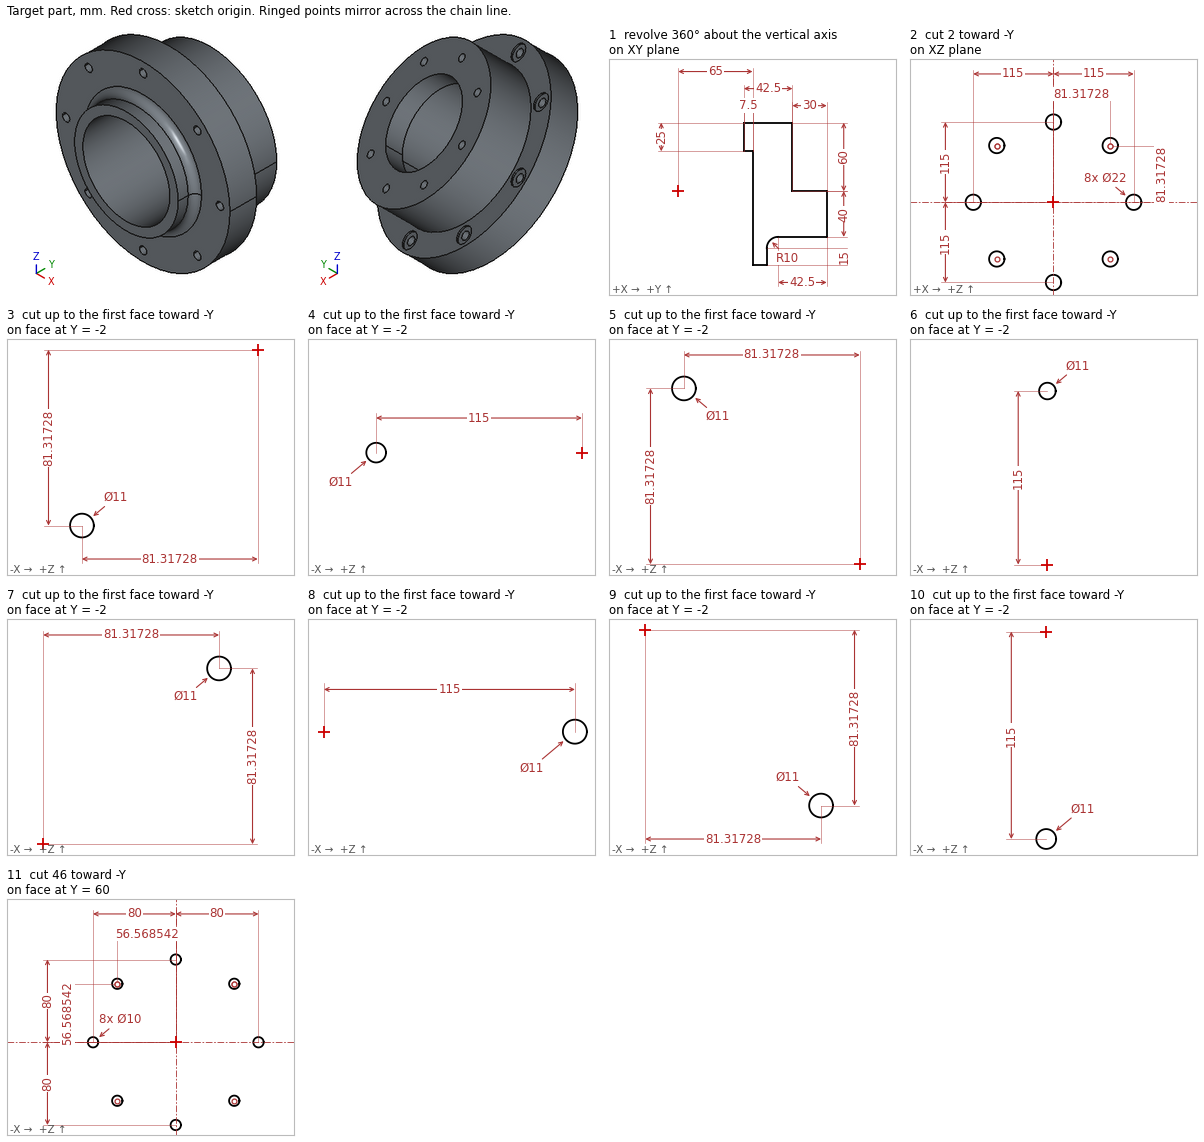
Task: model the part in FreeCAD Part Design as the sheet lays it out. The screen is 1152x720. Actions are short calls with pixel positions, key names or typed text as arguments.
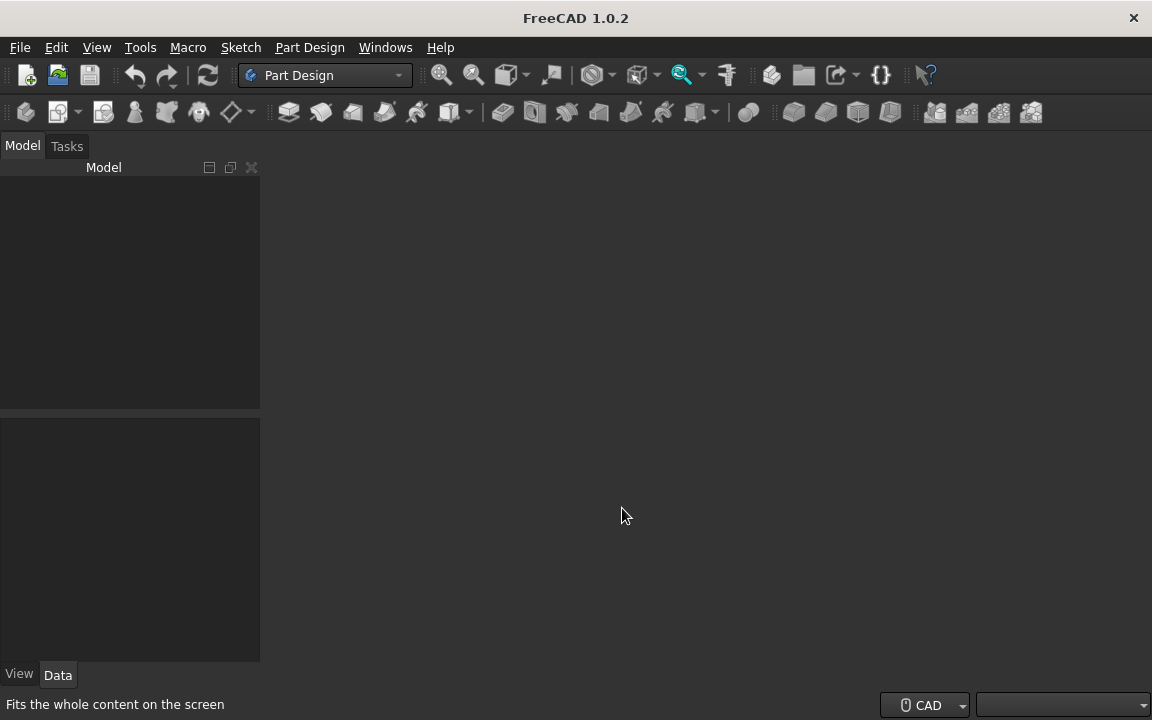
click(26, 76)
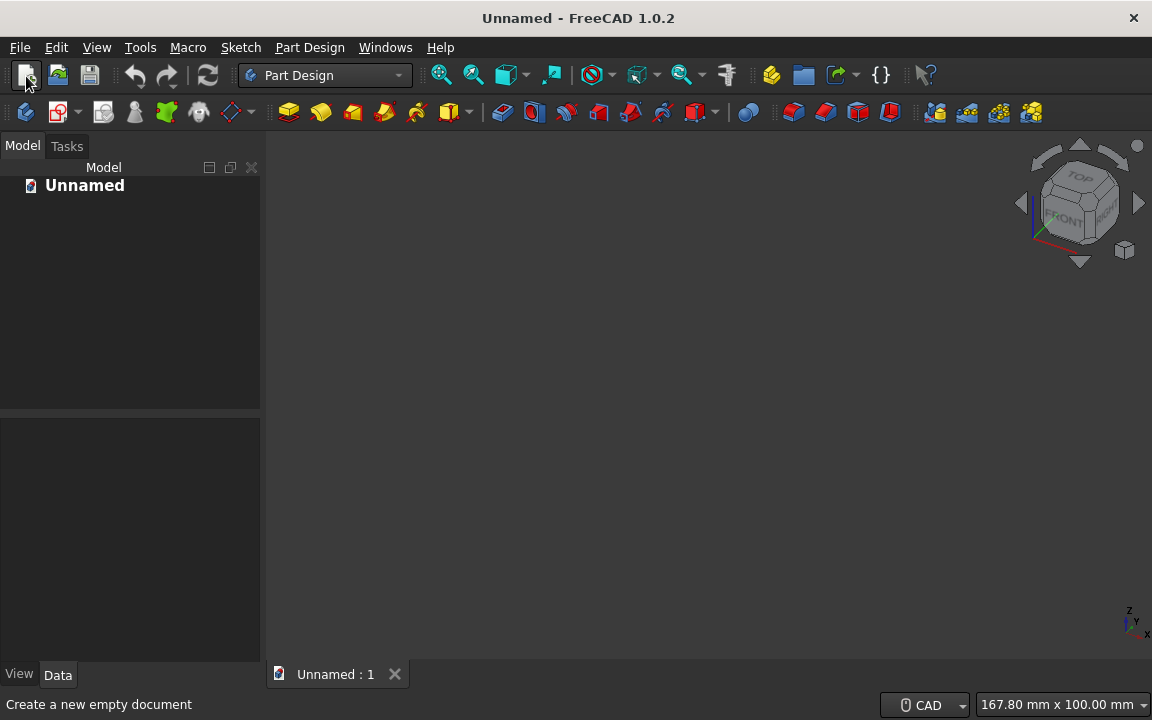
click(58, 112)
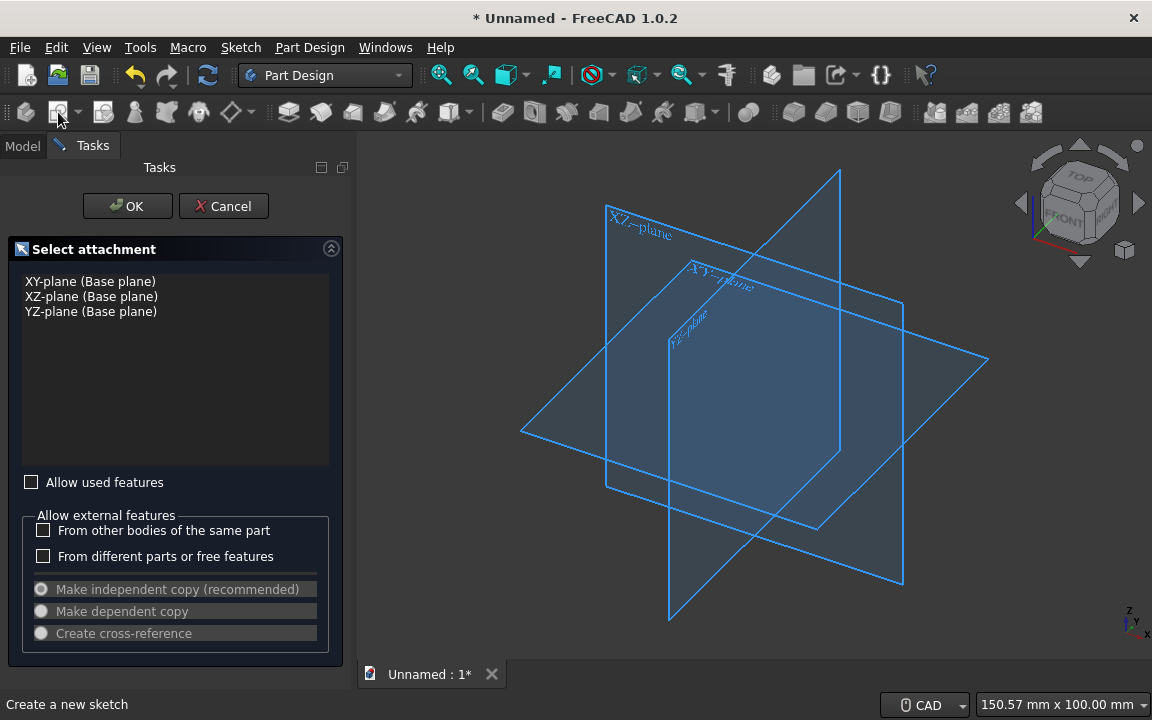
click(82, 282)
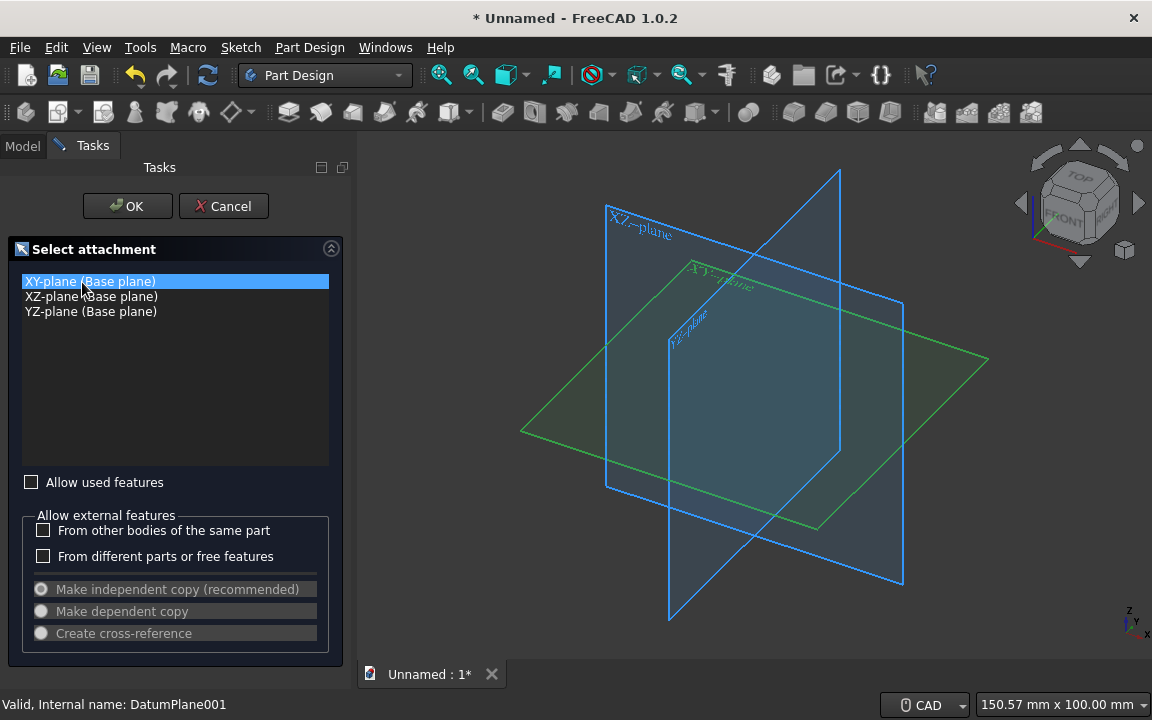
click(128, 206)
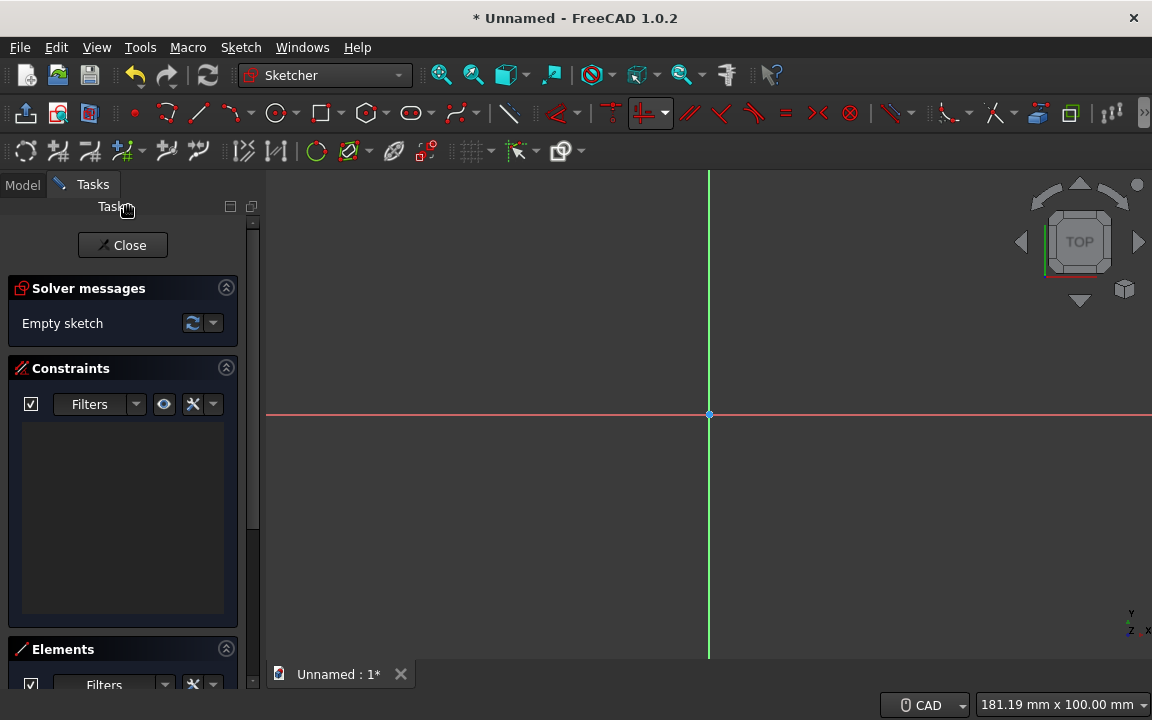
scroll(294, 400, down, 3)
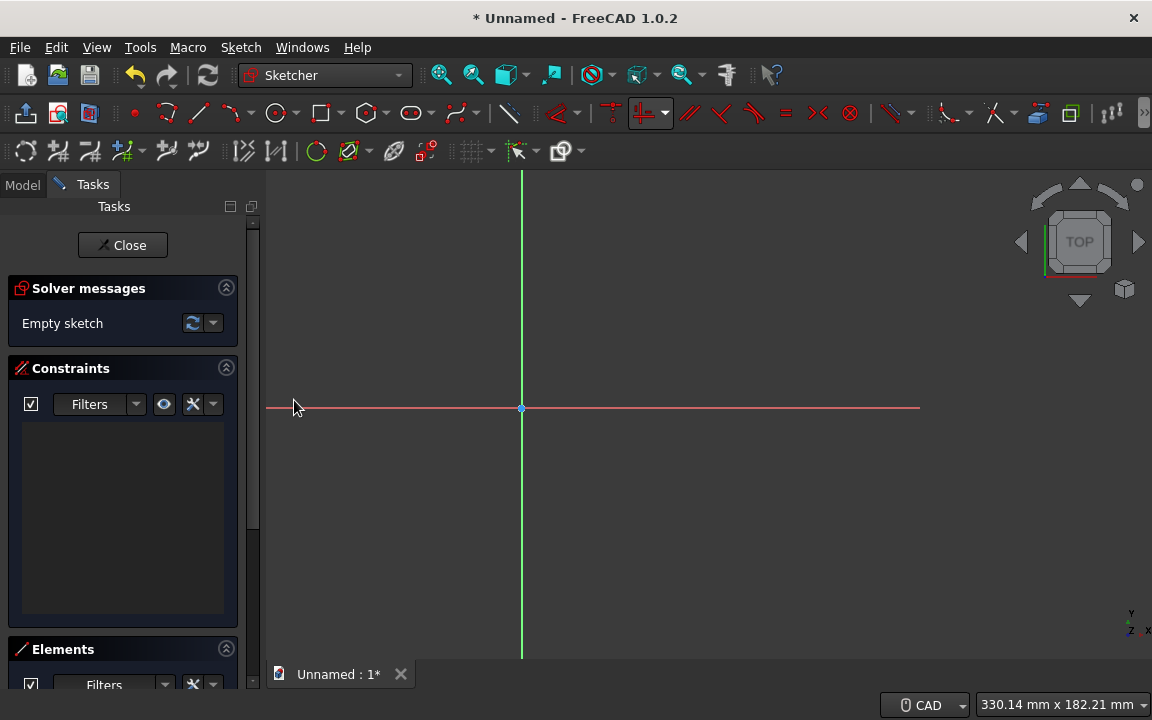
click(168, 114)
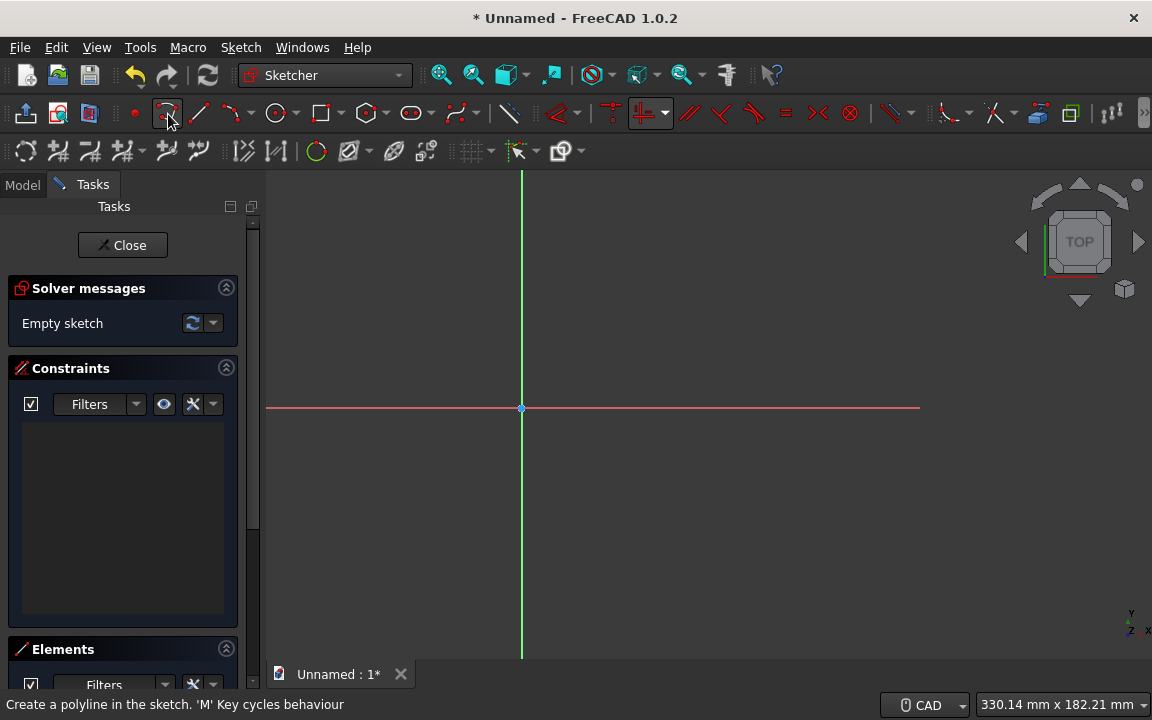
click(757, 516)
click(871, 516)
click(871, 408)
click(790, 417)
click(790, 247)
click(676, 247)
click(676, 314)
click(696, 314)
click(696, 583)
click(730, 583)
click(730, 542)
right_click(730, 542)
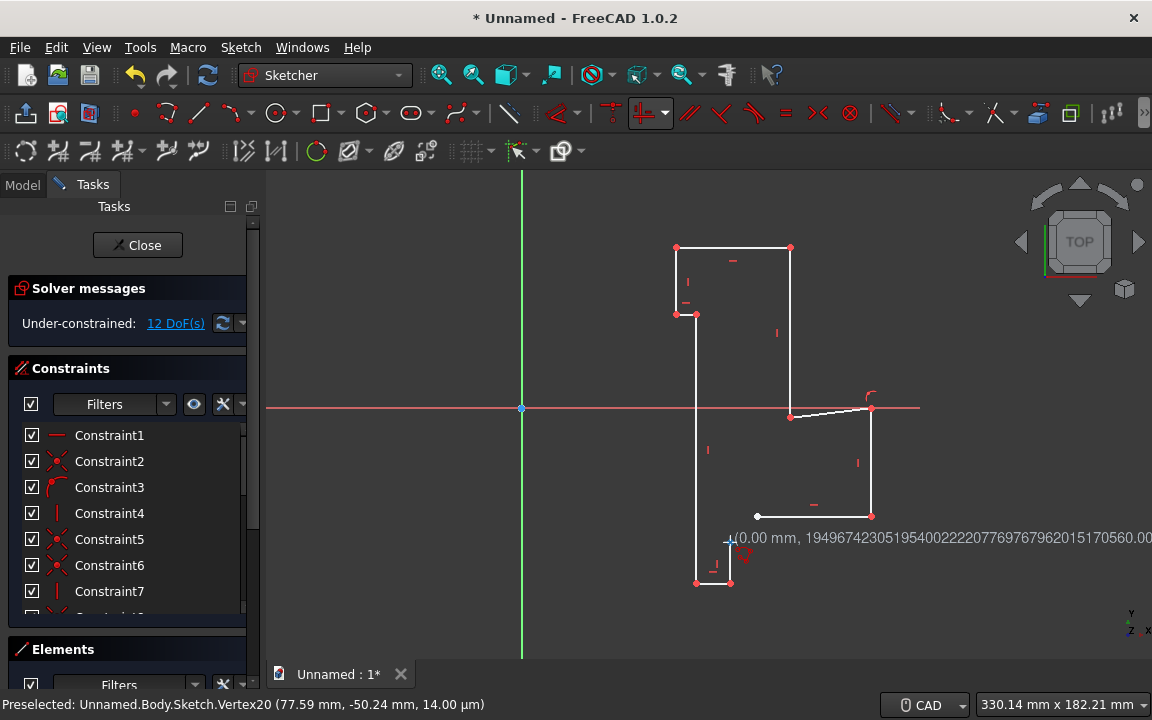
click(232, 114)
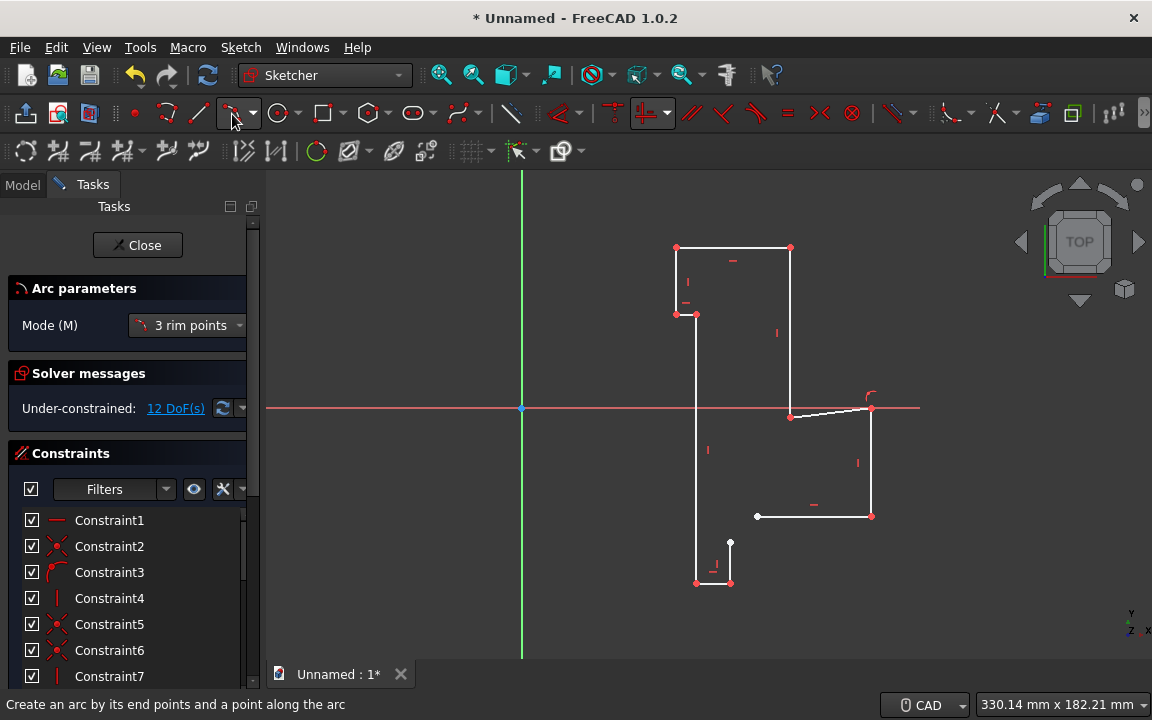
click(730, 543)
click(757, 517)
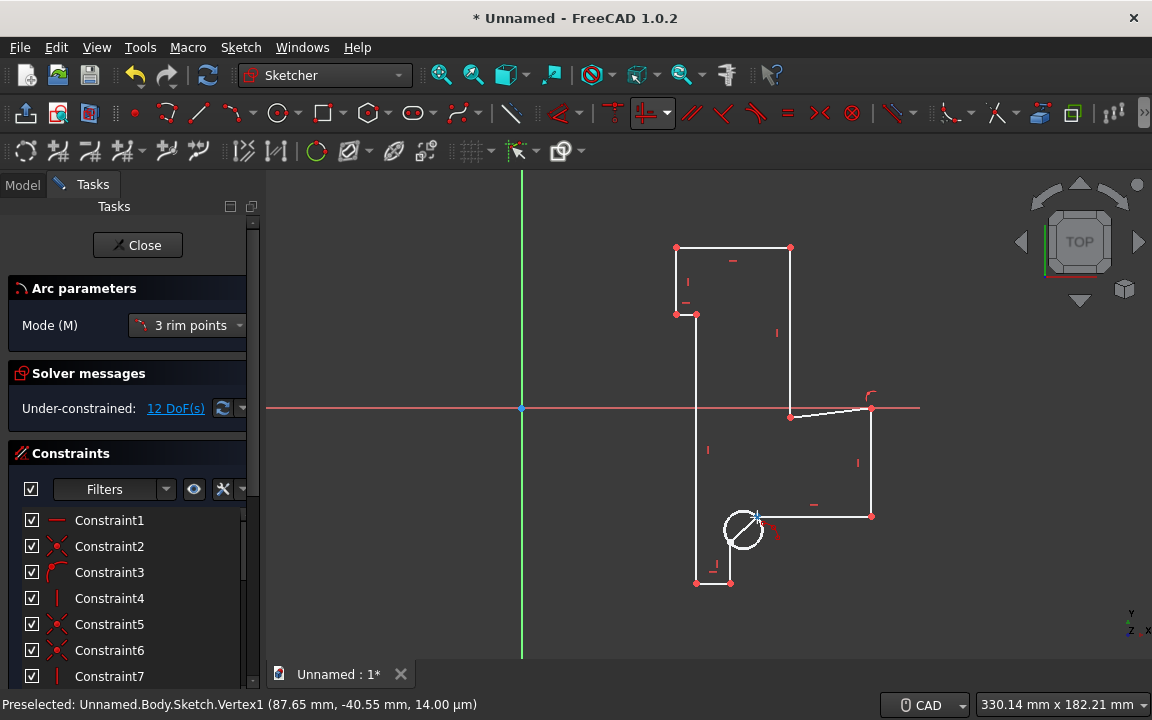
scroll(738, 523, up, 4)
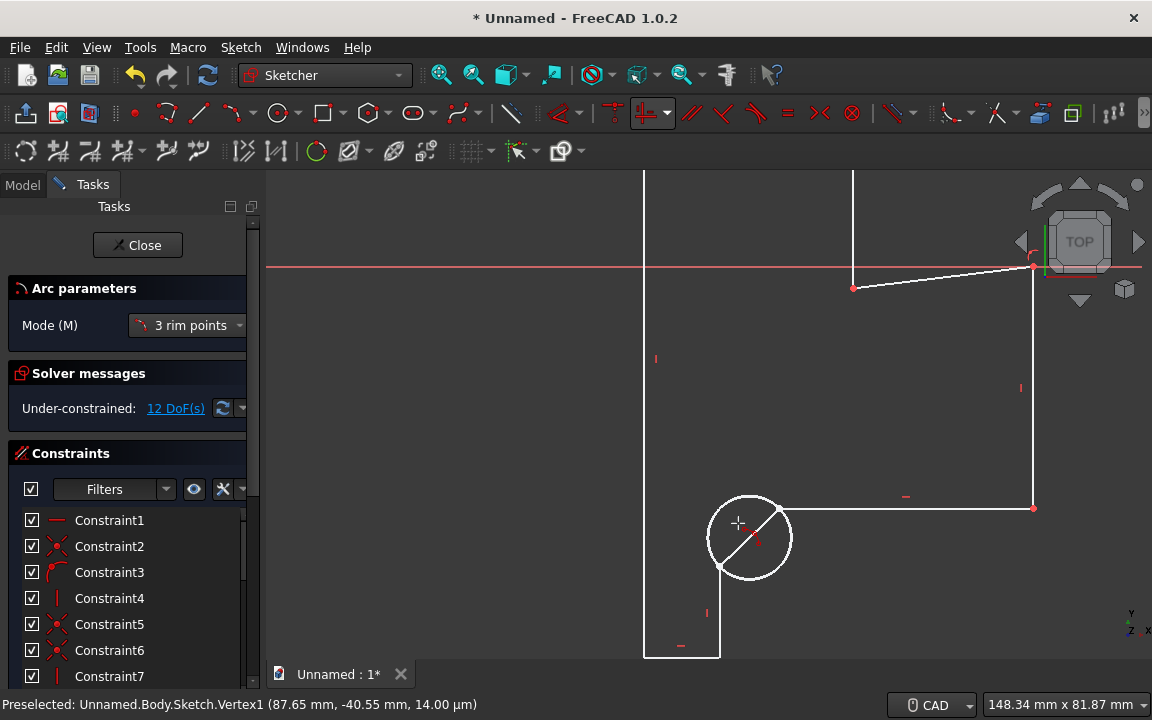
click(736, 523)
key(Escape)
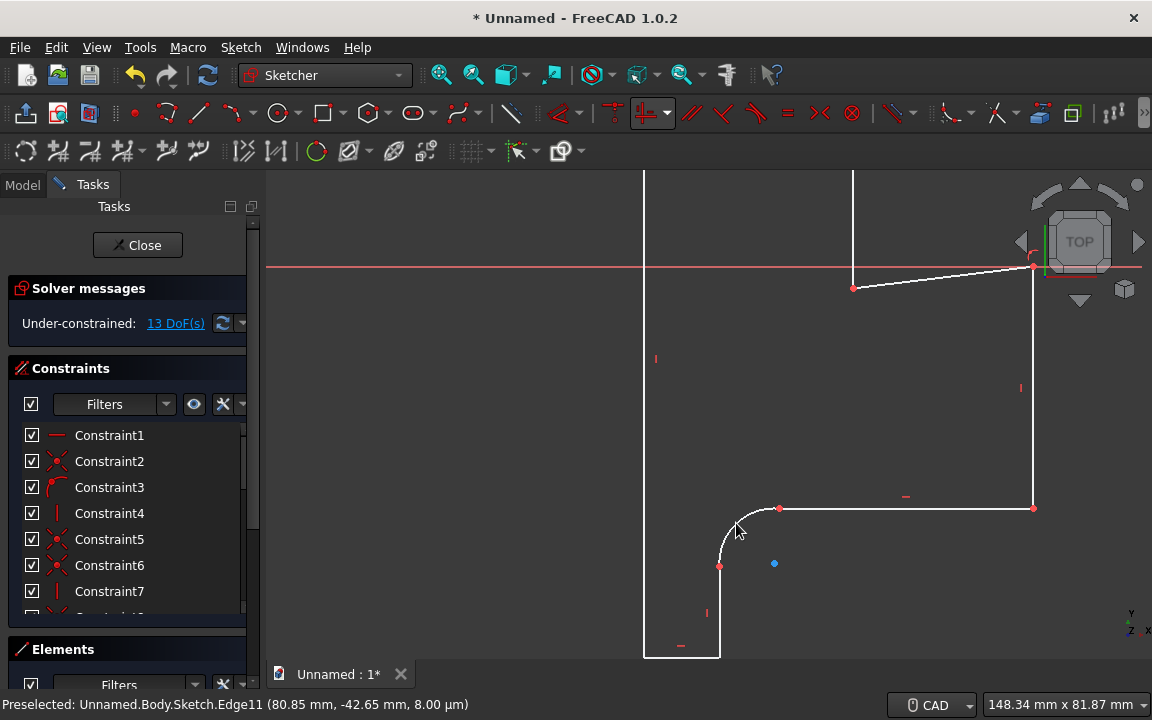
click(856, 509)